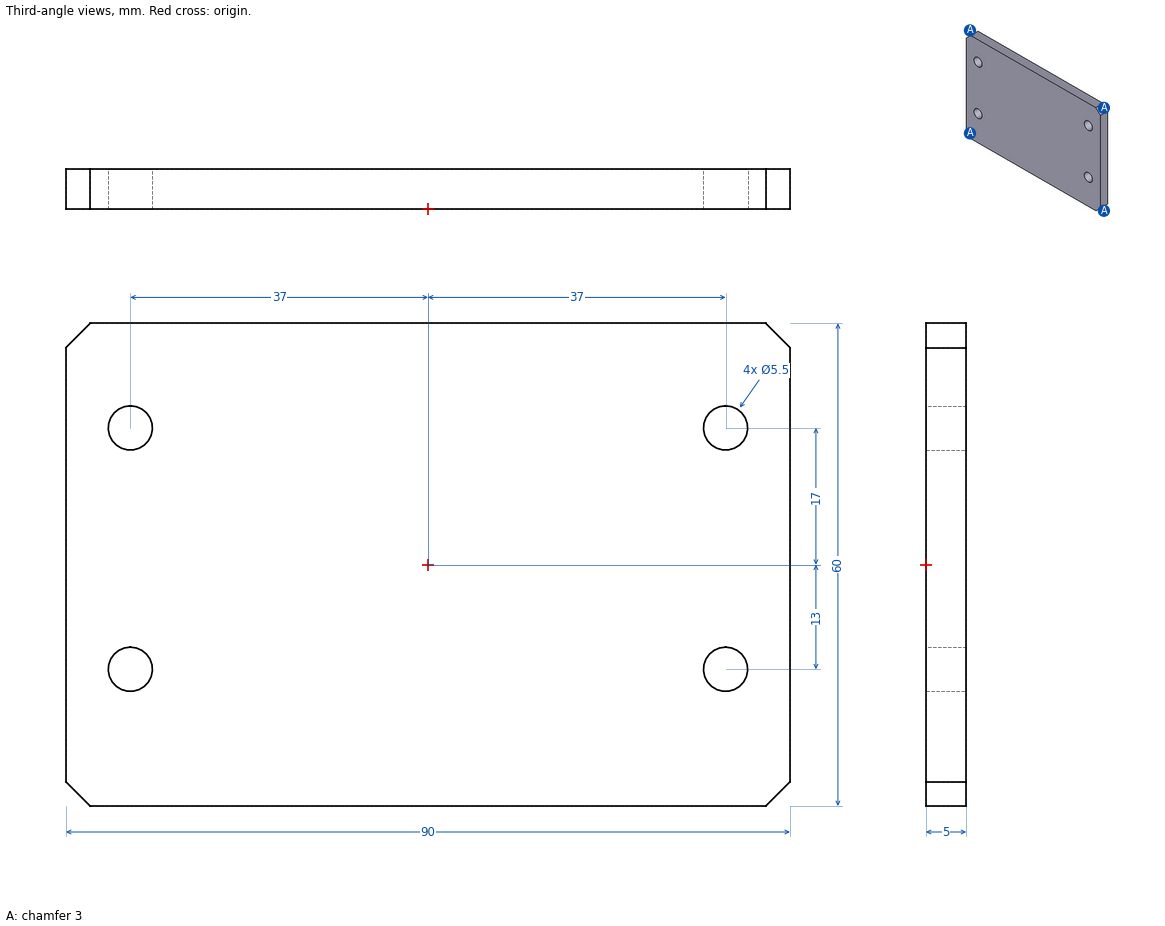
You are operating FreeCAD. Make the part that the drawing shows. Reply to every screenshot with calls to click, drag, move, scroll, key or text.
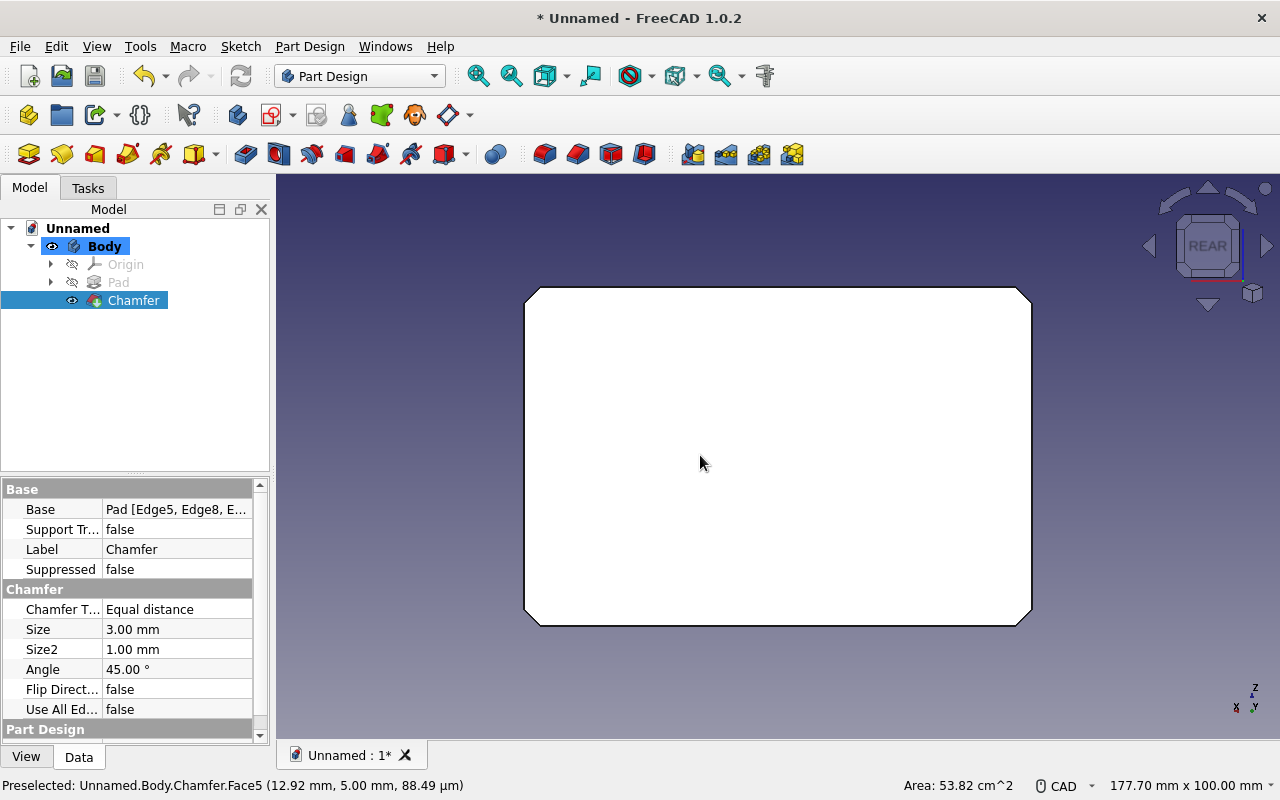
click(270, 116)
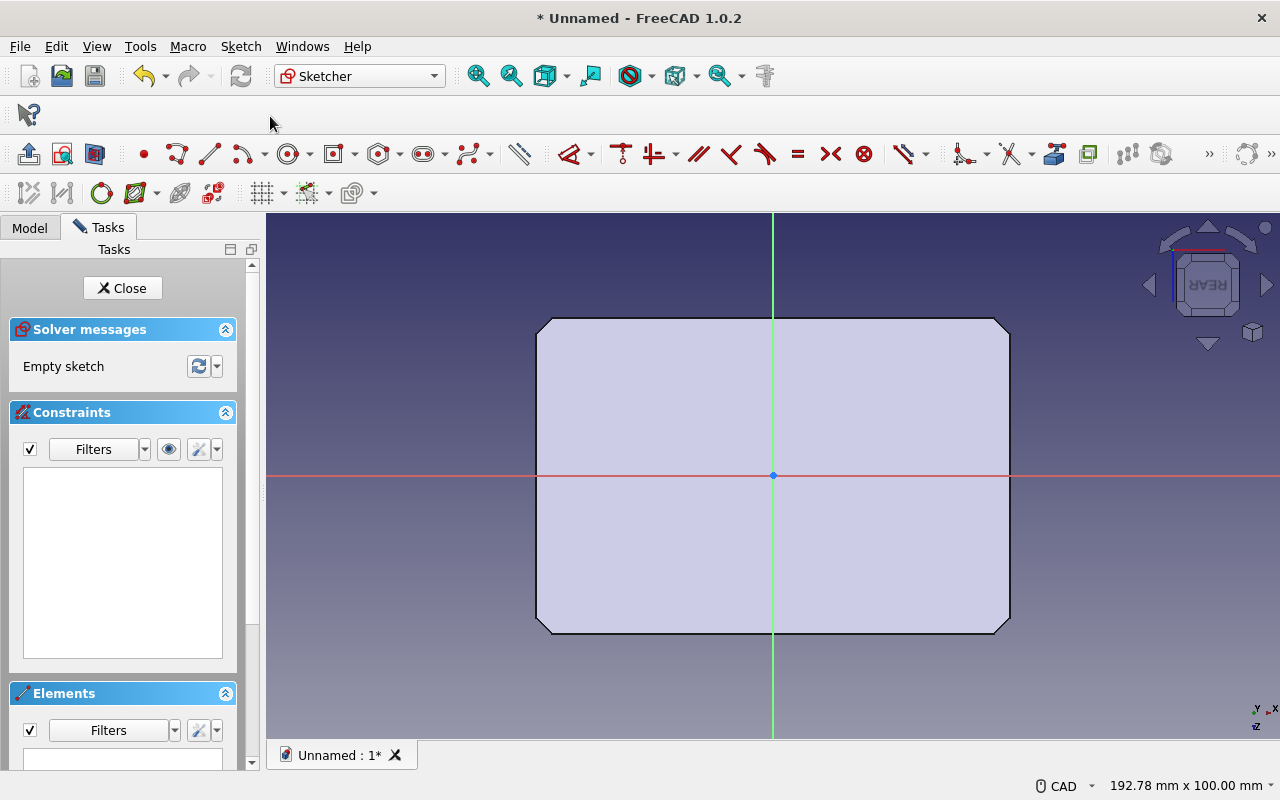
scroll(912, 508, up, 2)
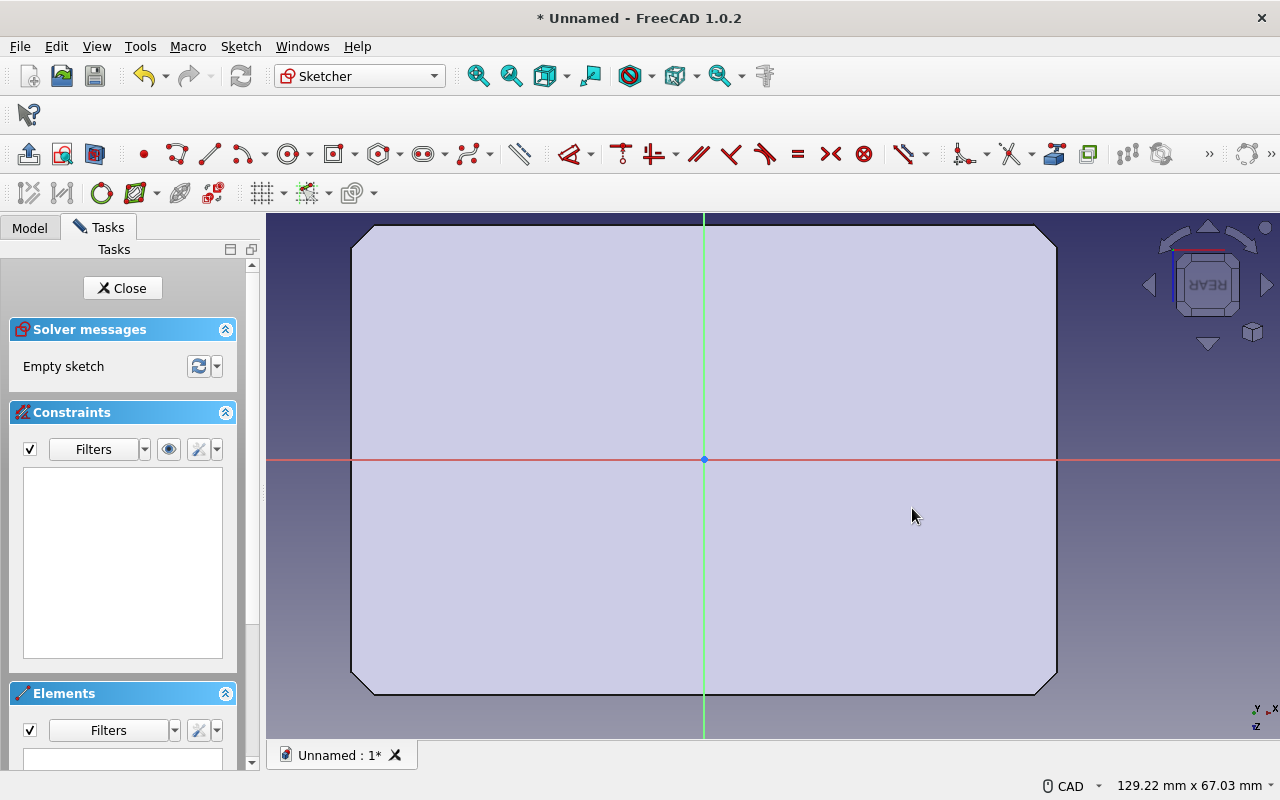
click(288, 154)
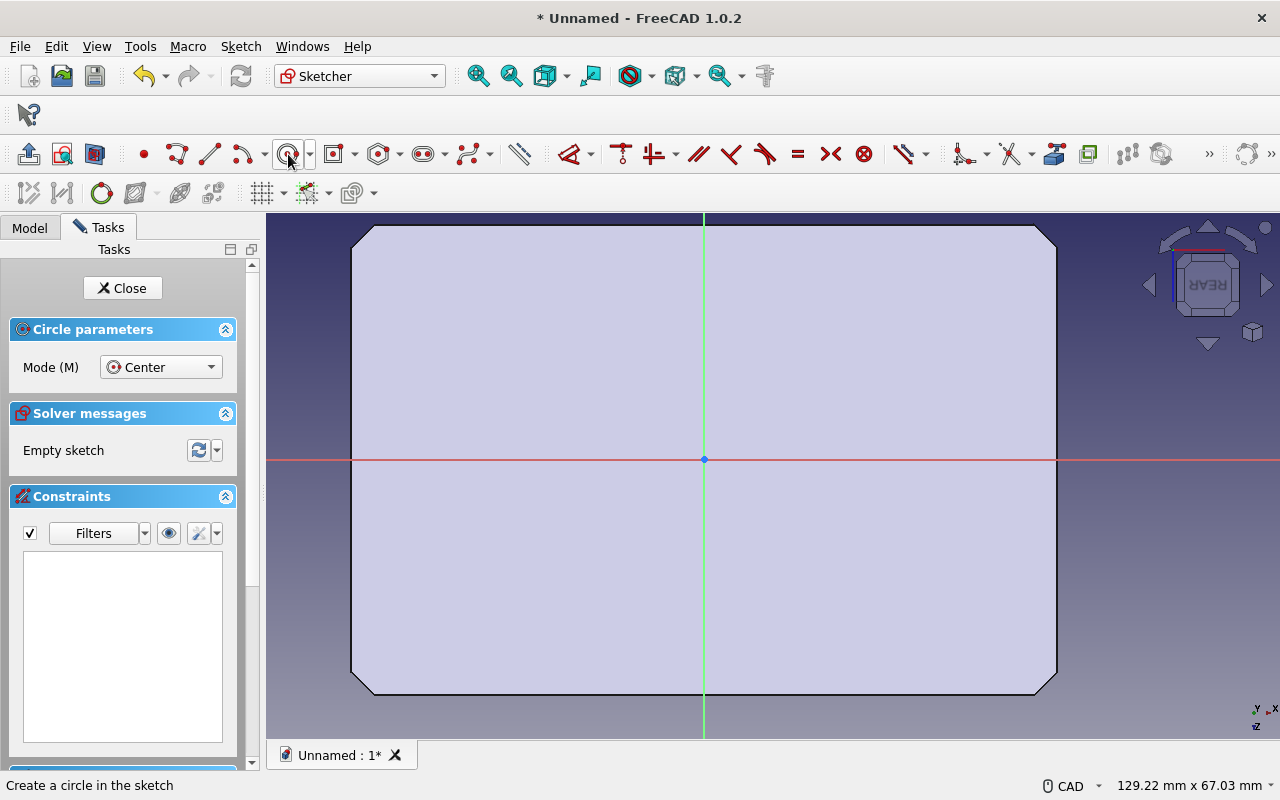
click(995, 593)
click(1010, 578)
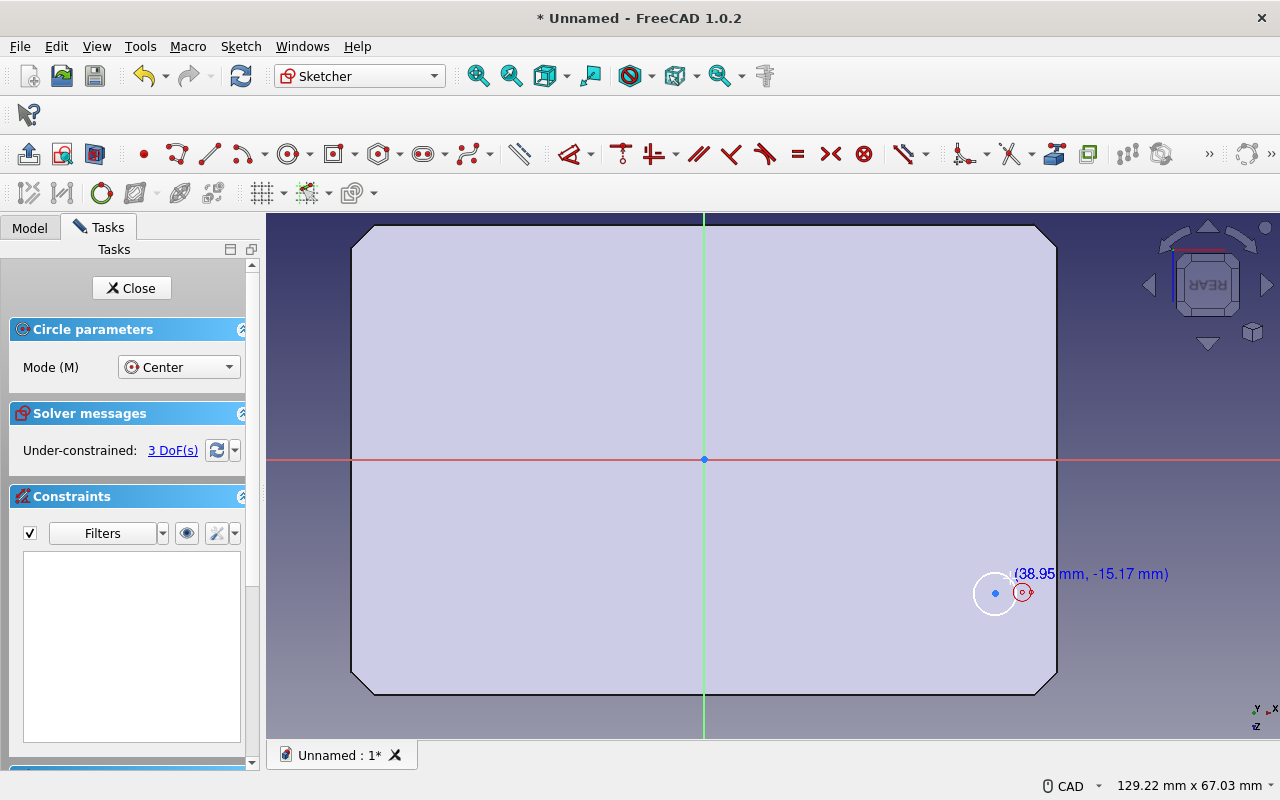
click(414, 593)
click(429, 578)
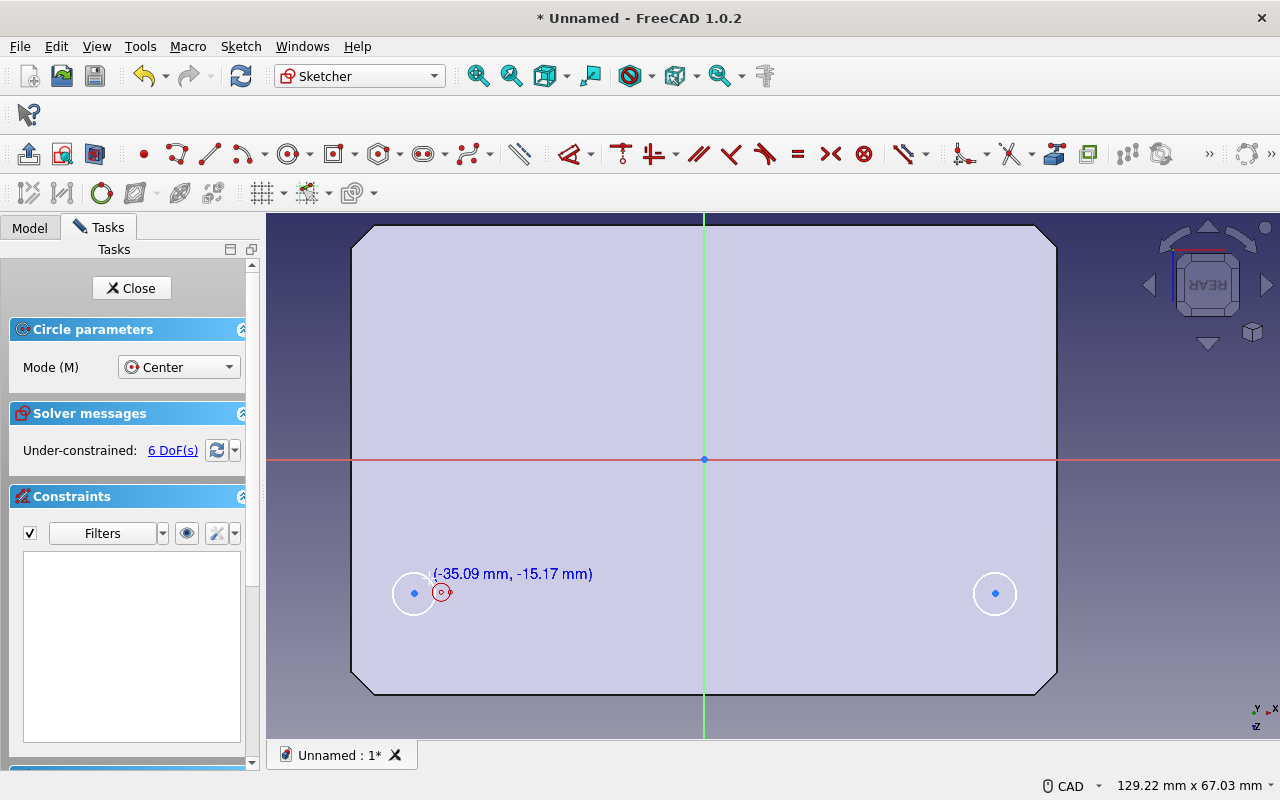
click(995, 358)
click(1010, 343)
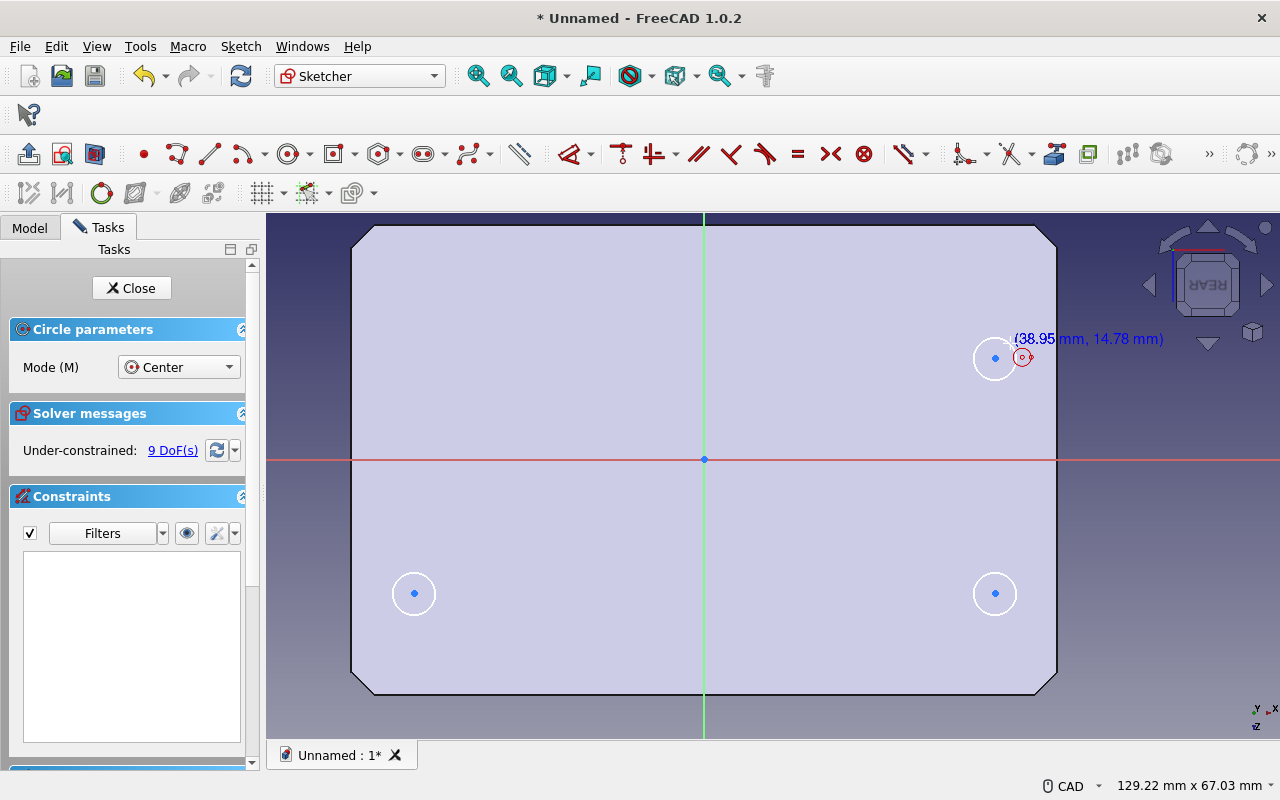
click(414, 358)
click(429, 343)
key(Escape)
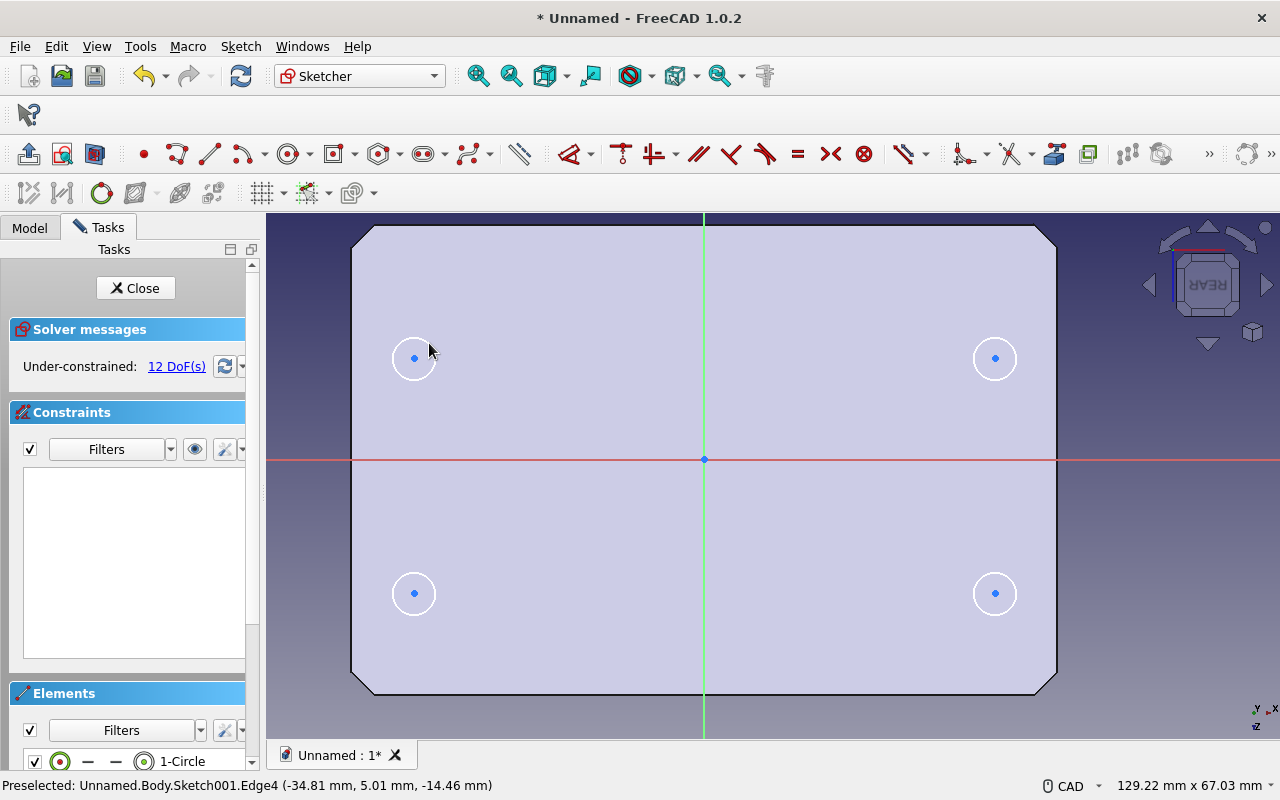
click(1010, 579)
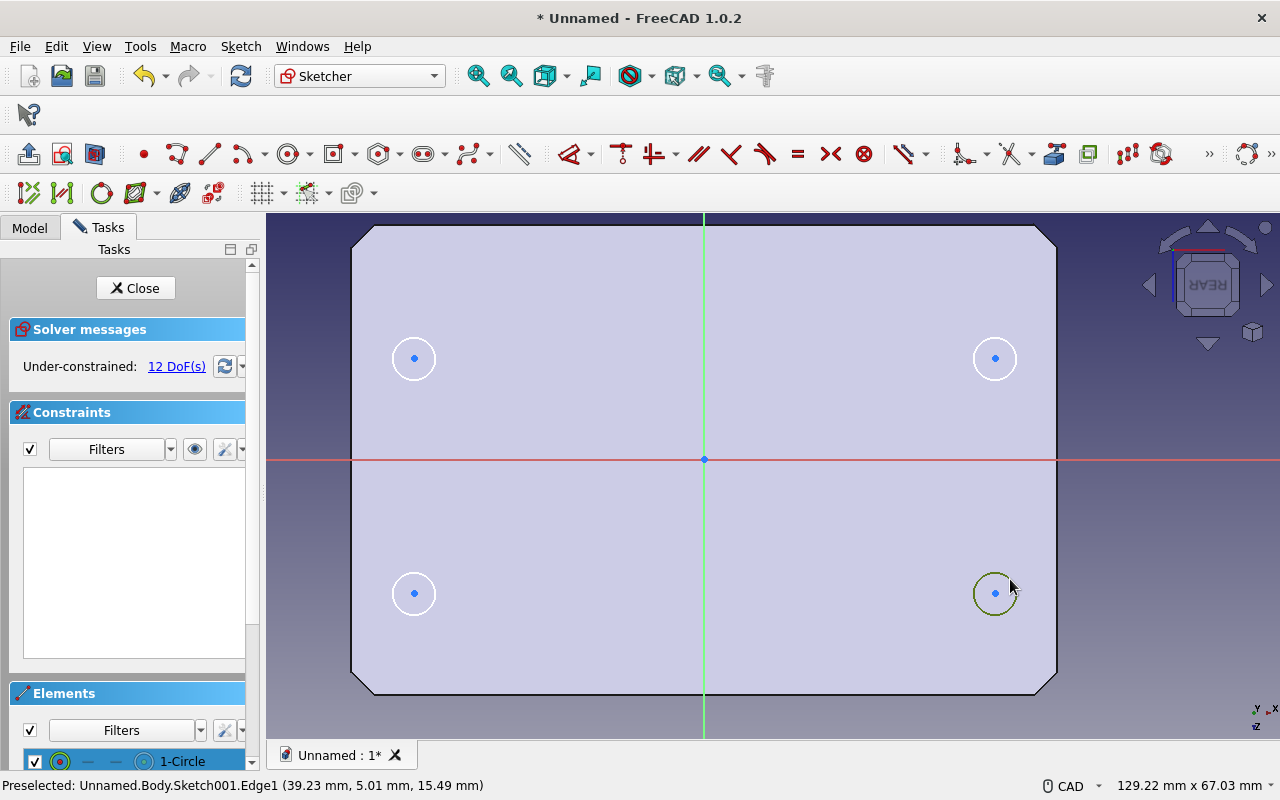
click(429, 579)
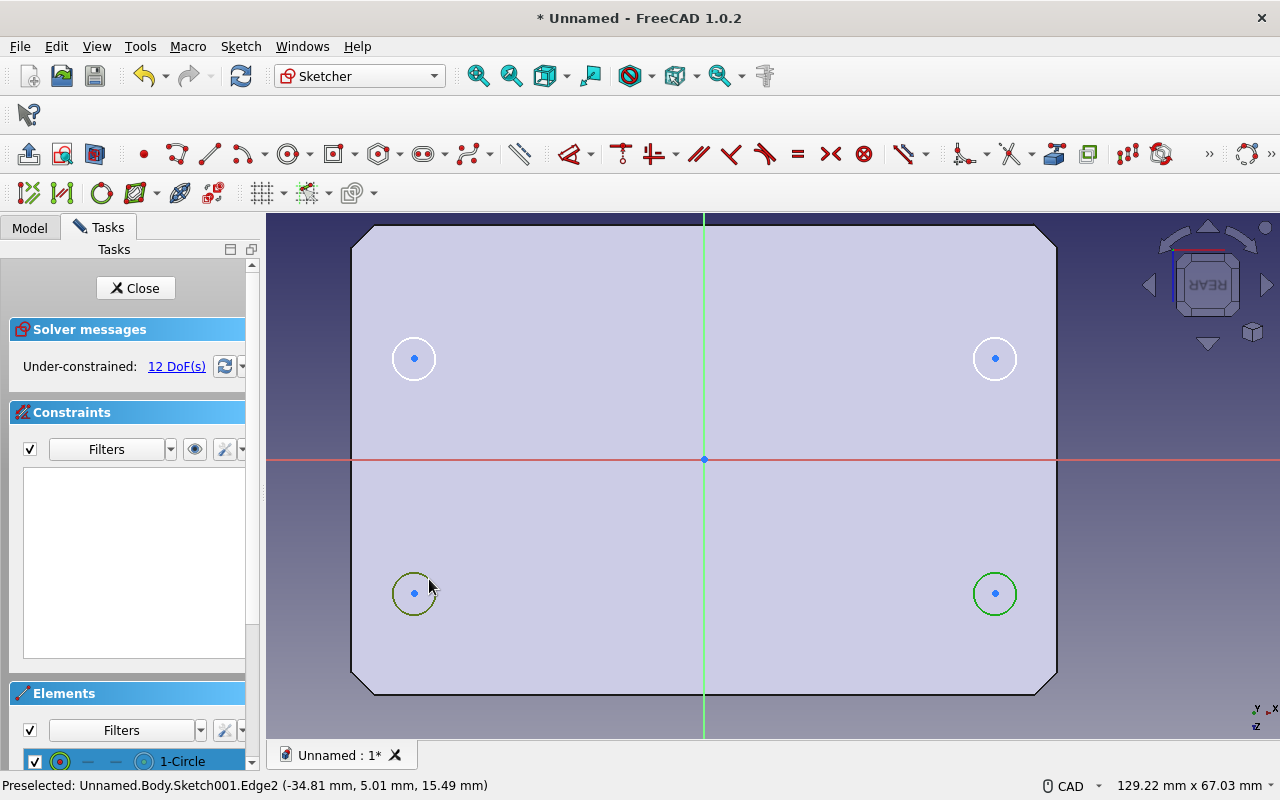
click(1010, 344)